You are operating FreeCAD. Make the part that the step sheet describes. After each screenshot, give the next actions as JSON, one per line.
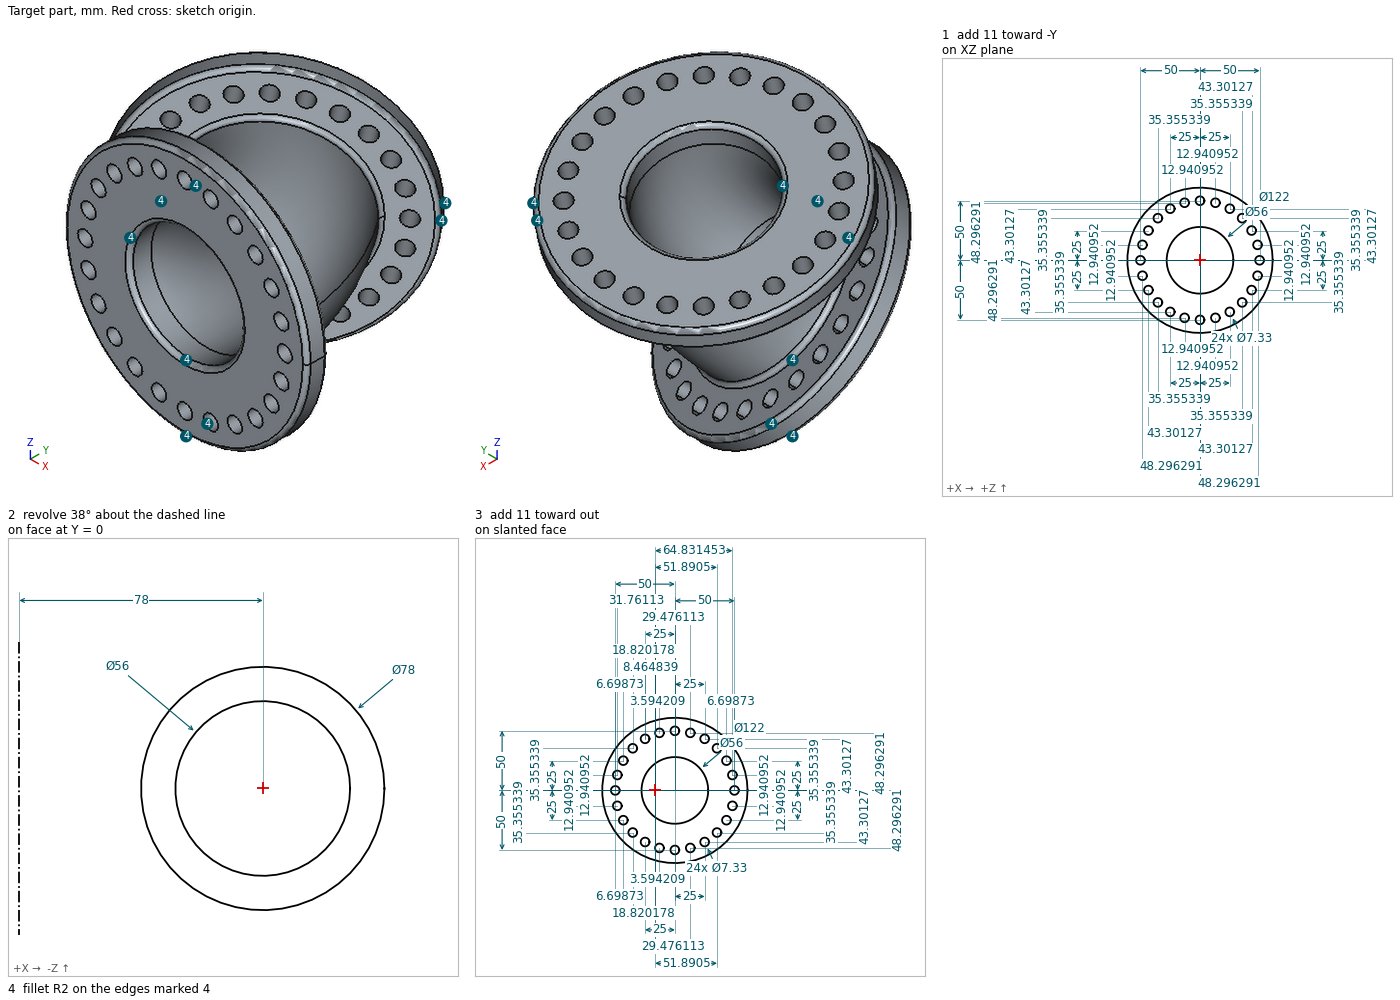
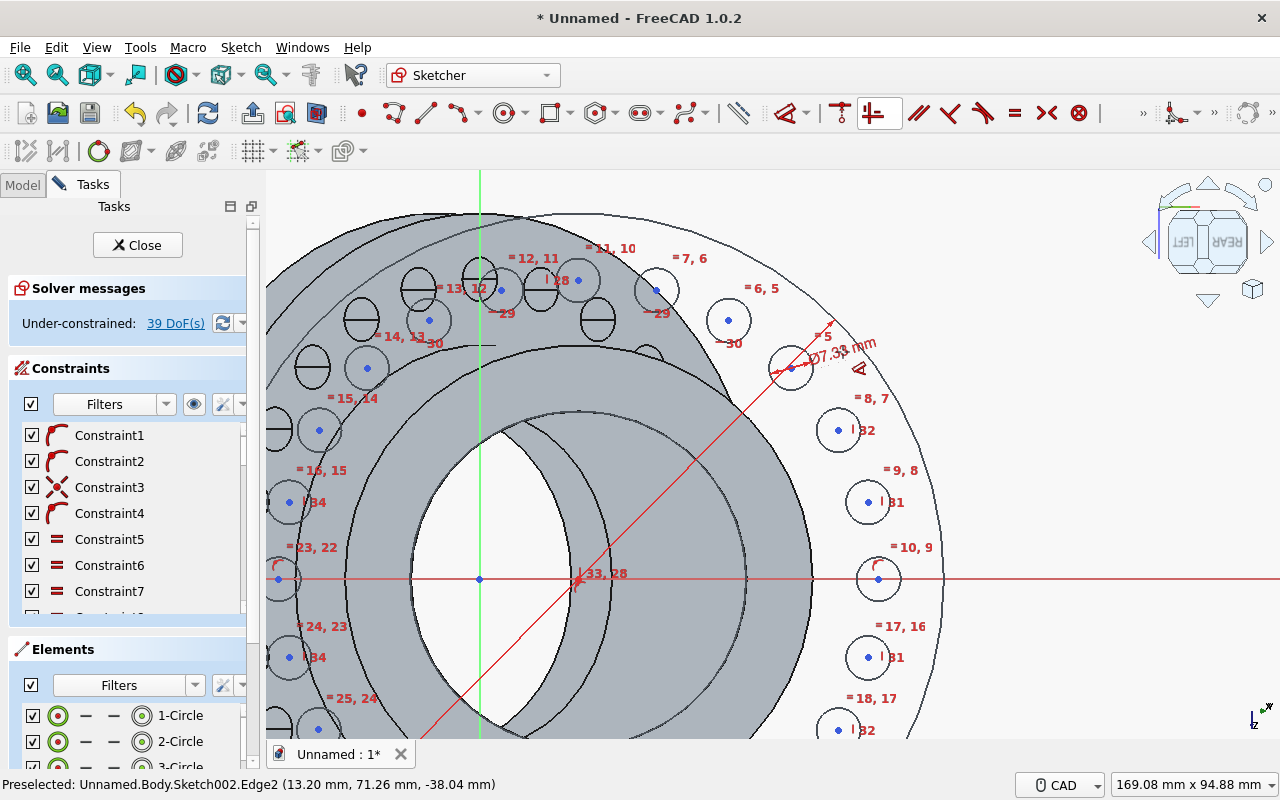
{"action": "left_click", "coordinate": [696, 460]}
{"action": "left_click", "coordinate": [719, 437]}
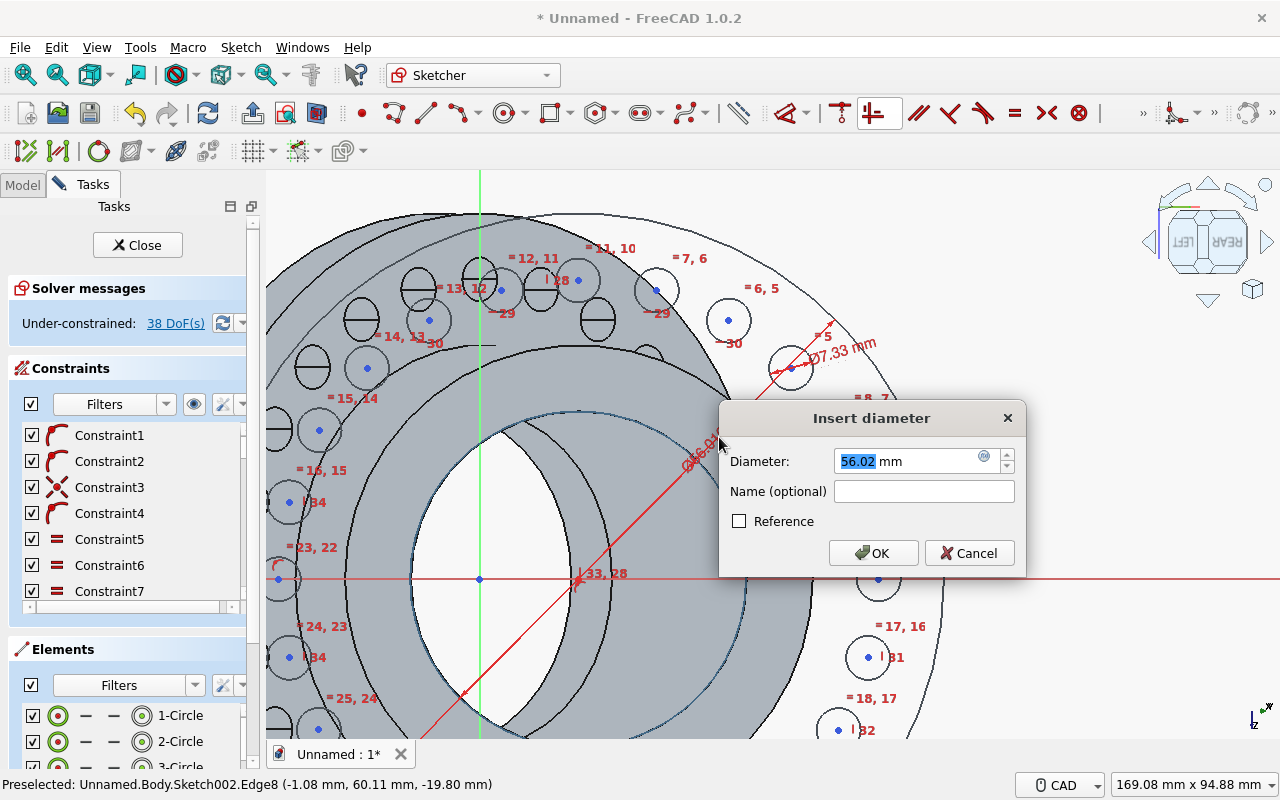
{"action": "type", "text": "56"}
{"action": "key", "text": "Return"}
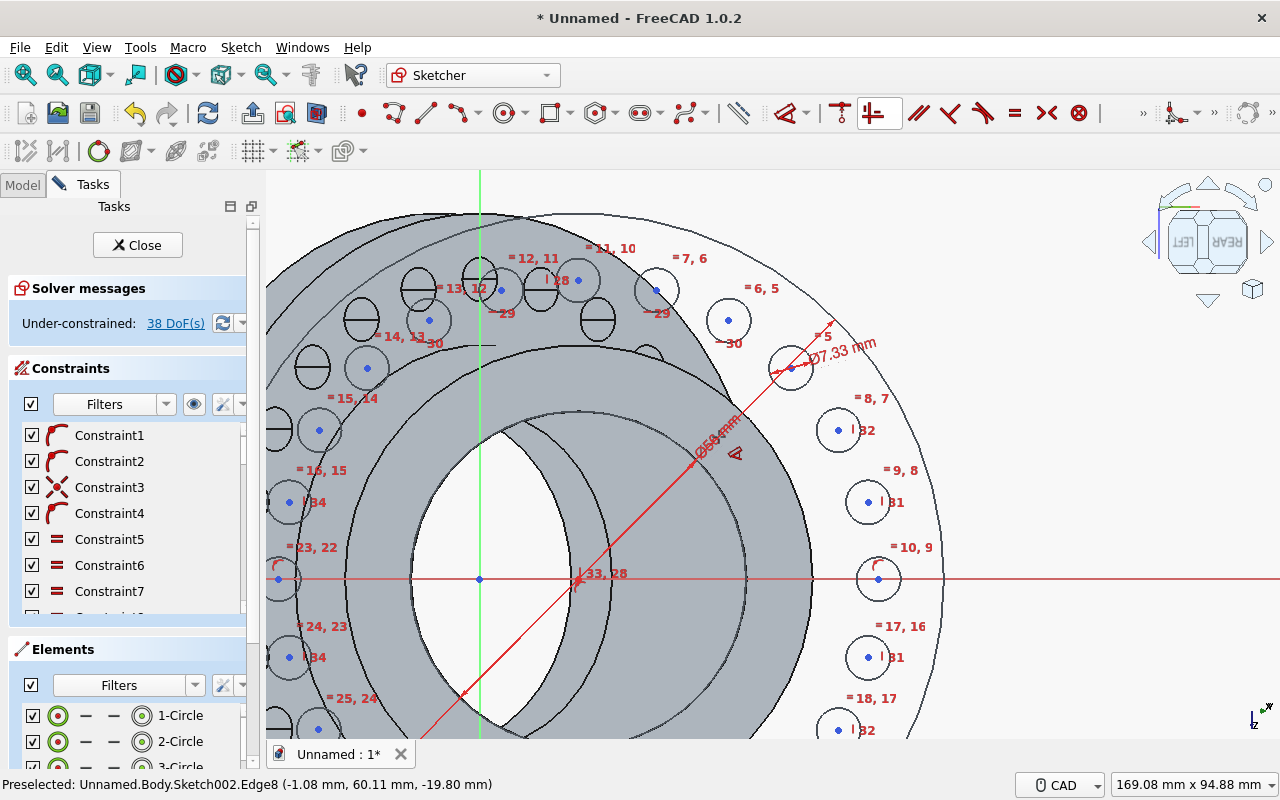
{"action": "left_click", "coordinate": [839, 430]}
{"action": "left_click", "coordinate": [873, 505]}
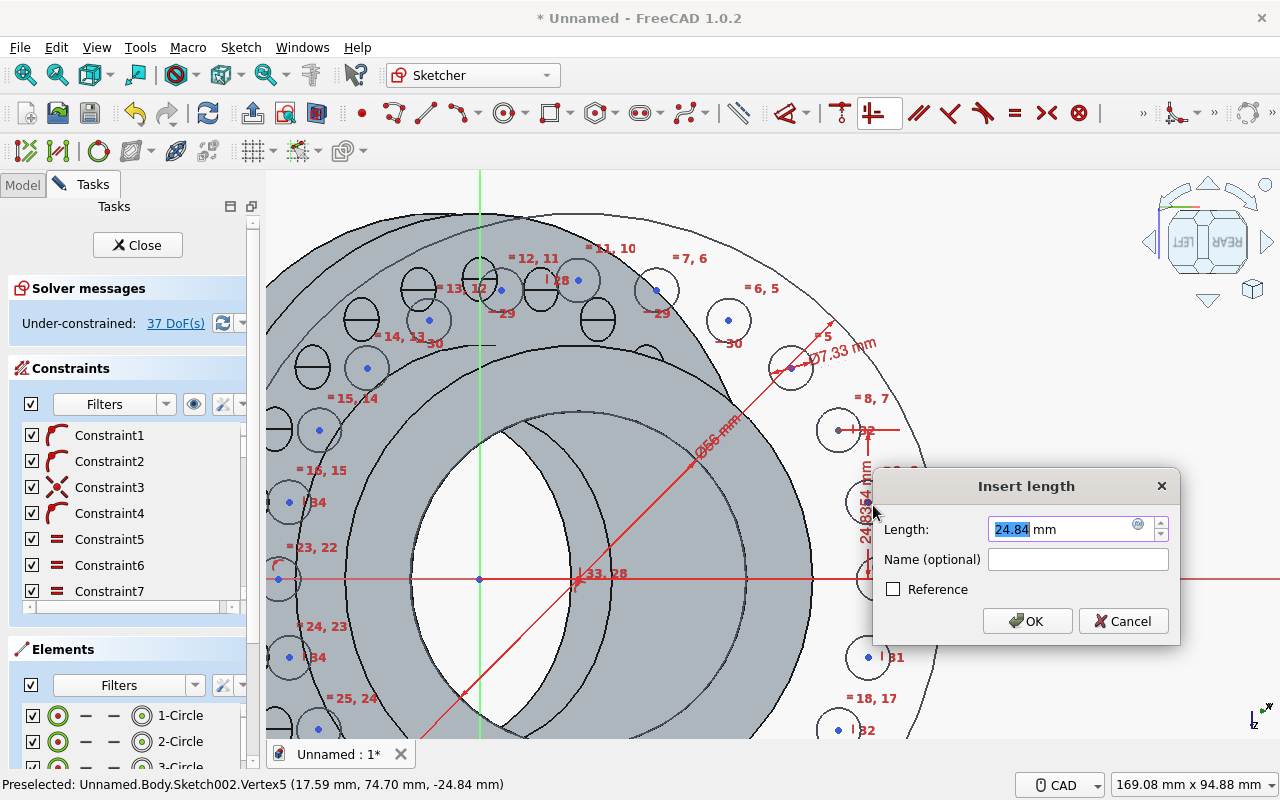
{"action": "type", "text": "25"}
{"action": "key", "text": "Return"}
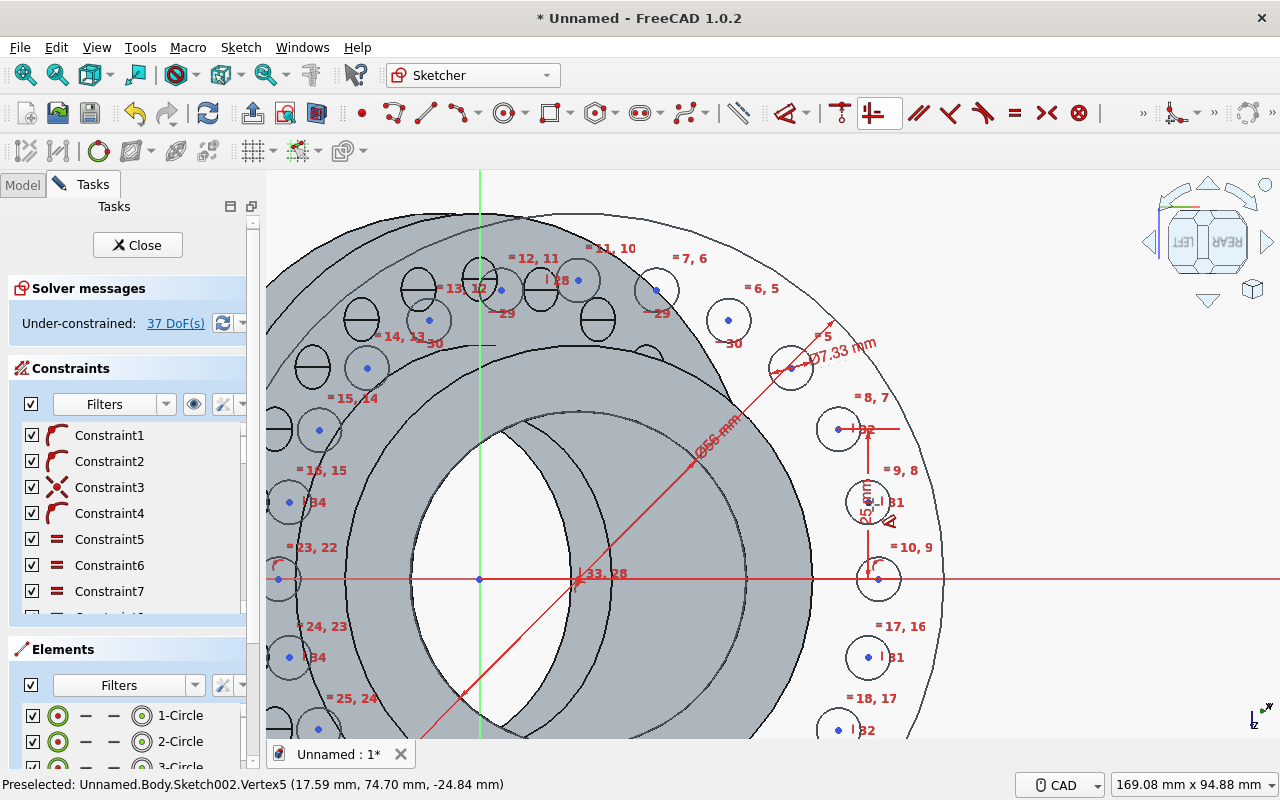
{"action": "left_click", "coordinate": [578, 280]}
{"action": "left_click", "coordinate": [446, 430]}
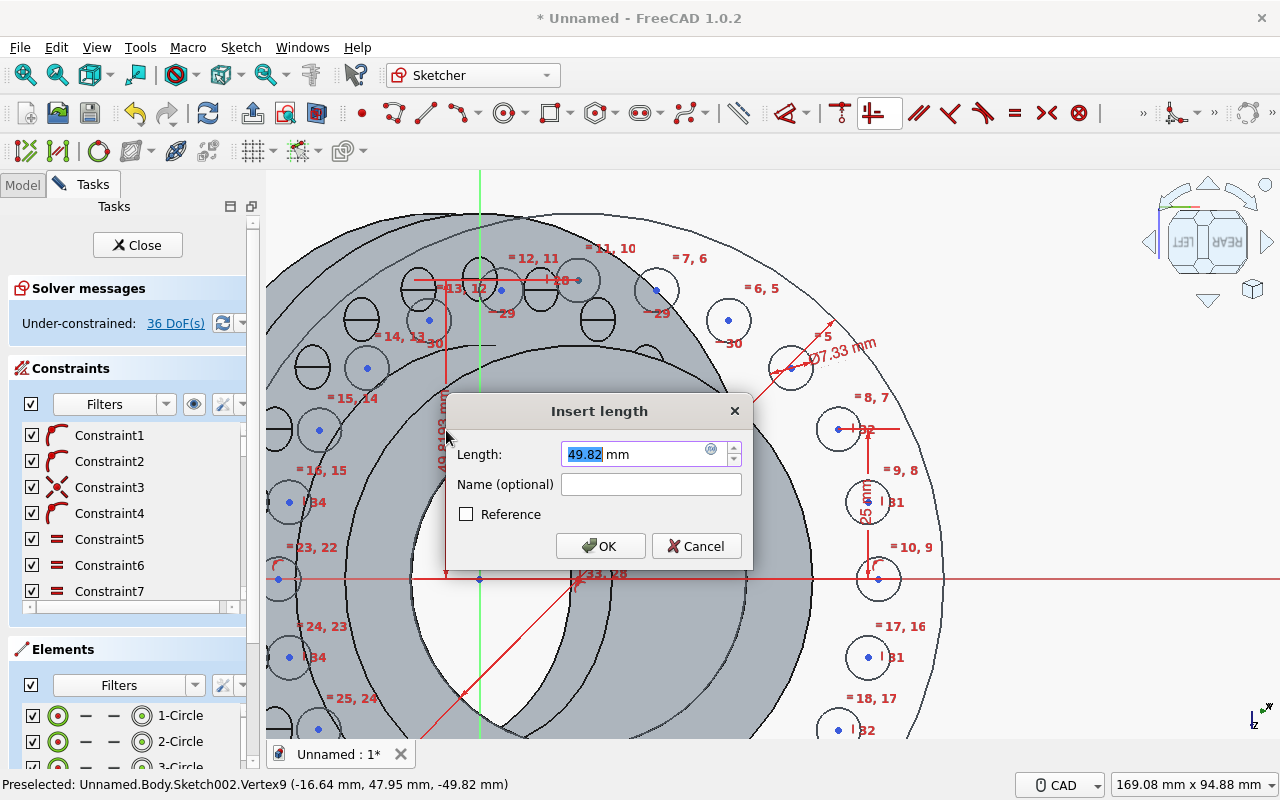
{"action": "type", "text": "50"}
{"action": "key", "text": "Return"}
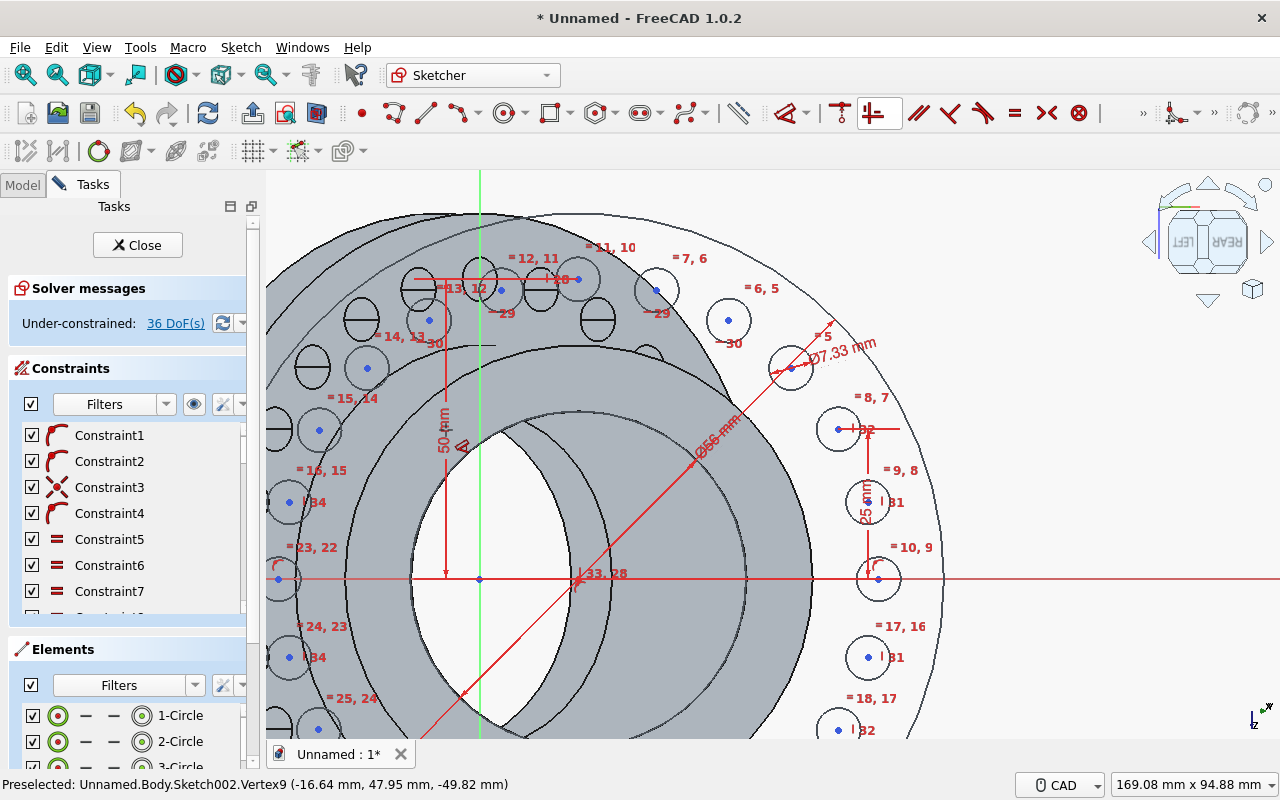
{"action": "left_click", "coordinate": [320, 430]}
{"action": "left_click", "coordinate": [514, 505]}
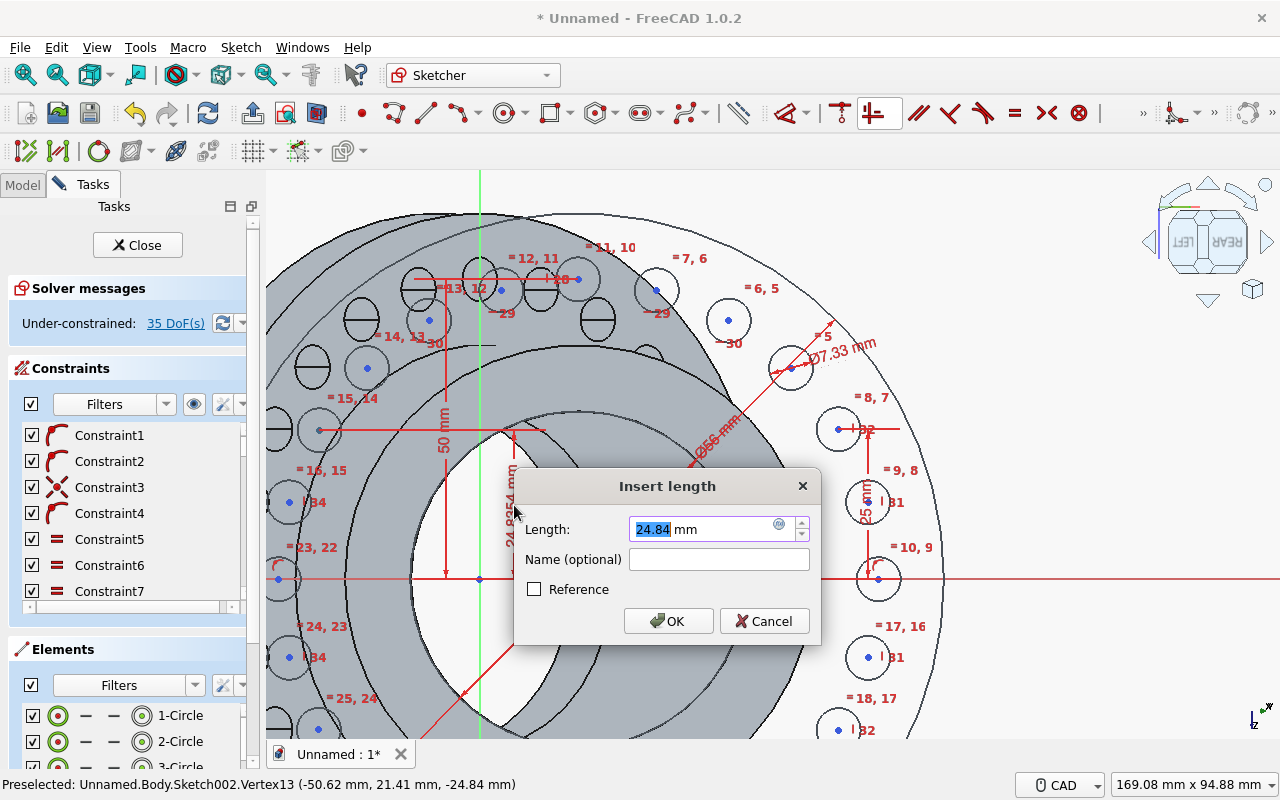
{"action": "type", "text": "25"}
{"action": "key", "text": "Return"}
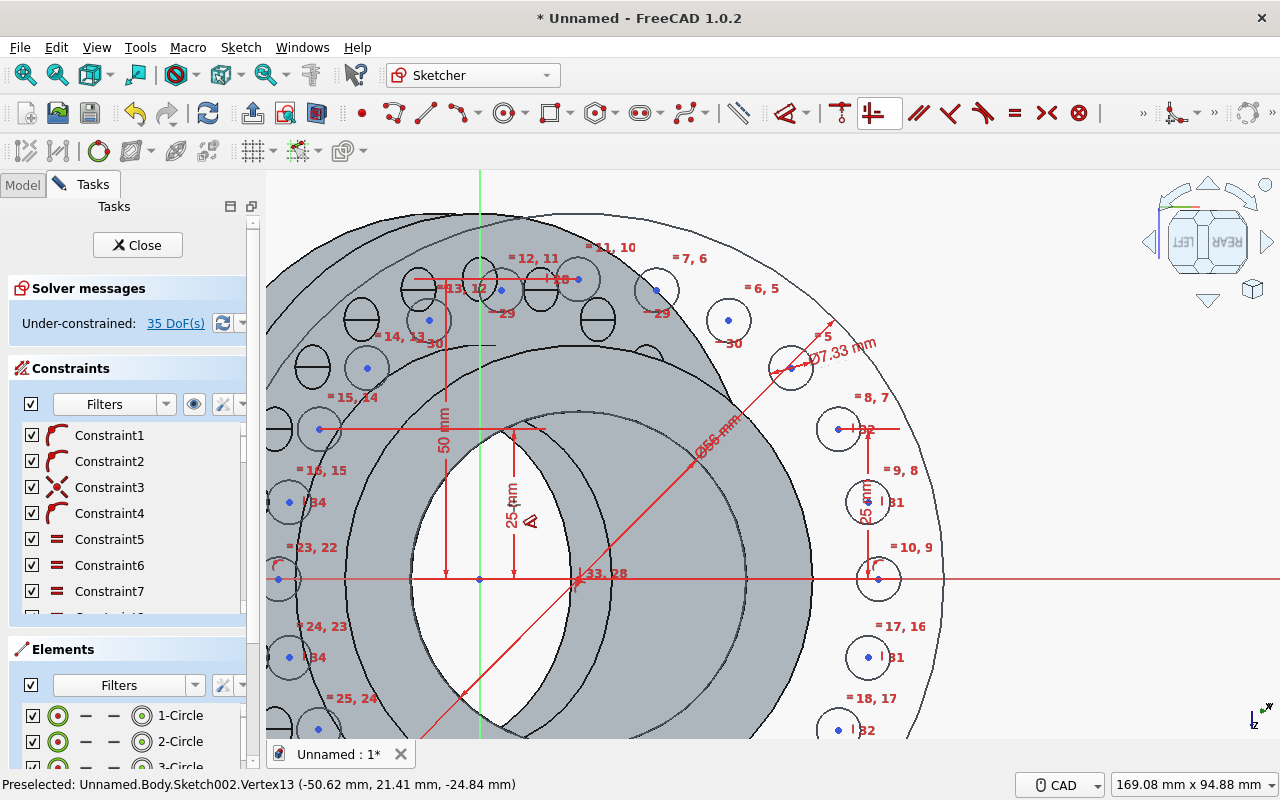
{"action": "scroll", "coordinate": [807, 353], "scroll_direction": "down", "scroll_amount": 4}